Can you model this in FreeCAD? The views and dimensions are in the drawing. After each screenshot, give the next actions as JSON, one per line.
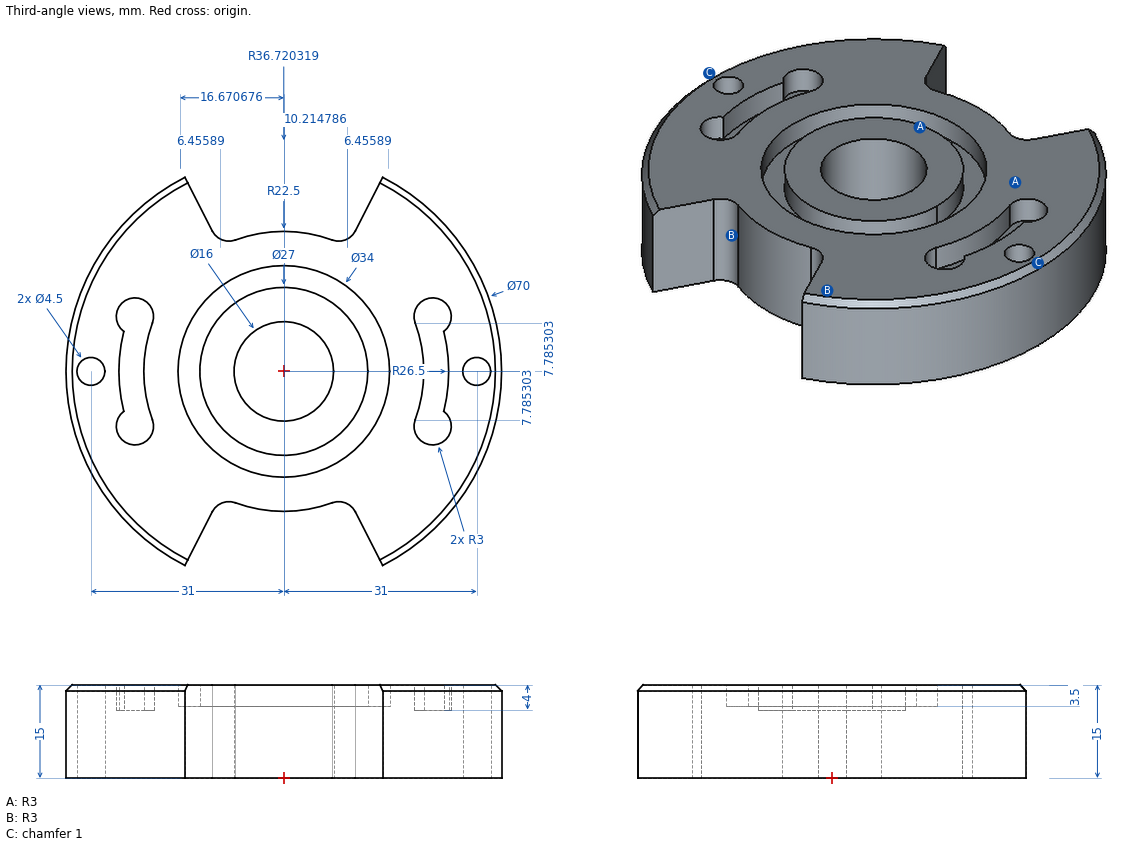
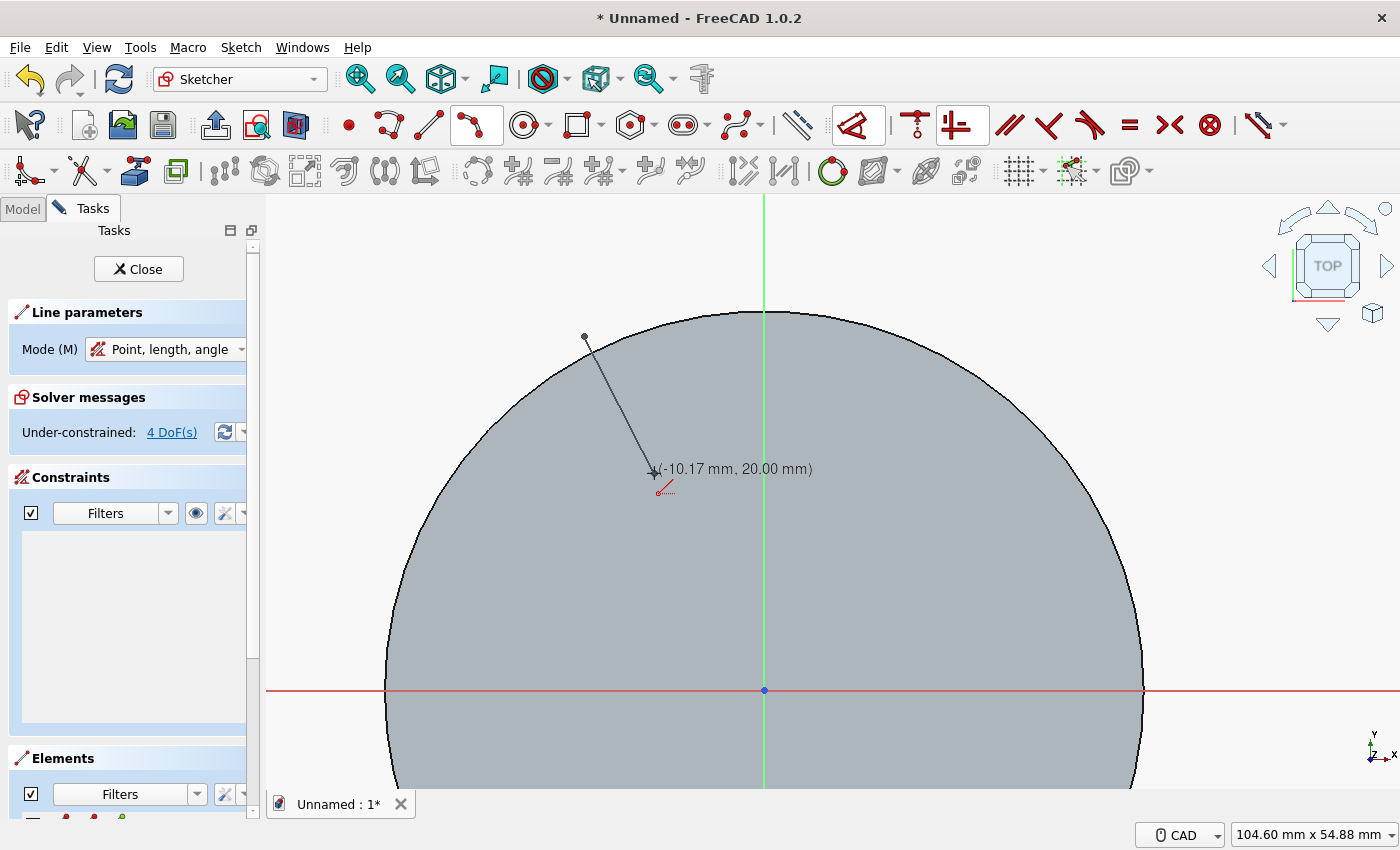
{"action": "left_click", "coordinate": [875, 473]}
{"action": "left_click", "coordinate": [945, 336]}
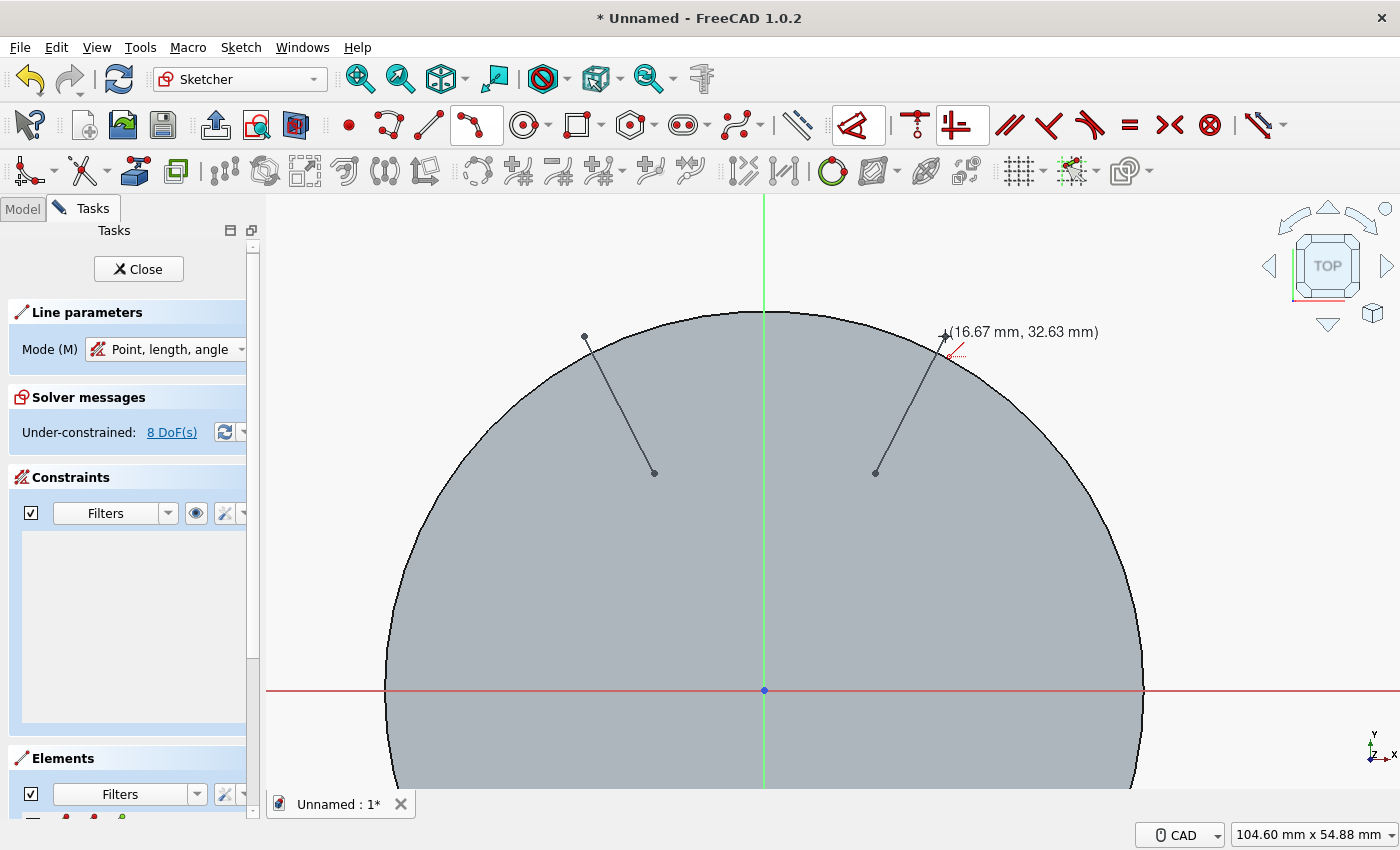
{"action": "key", "text": "g 3 a"}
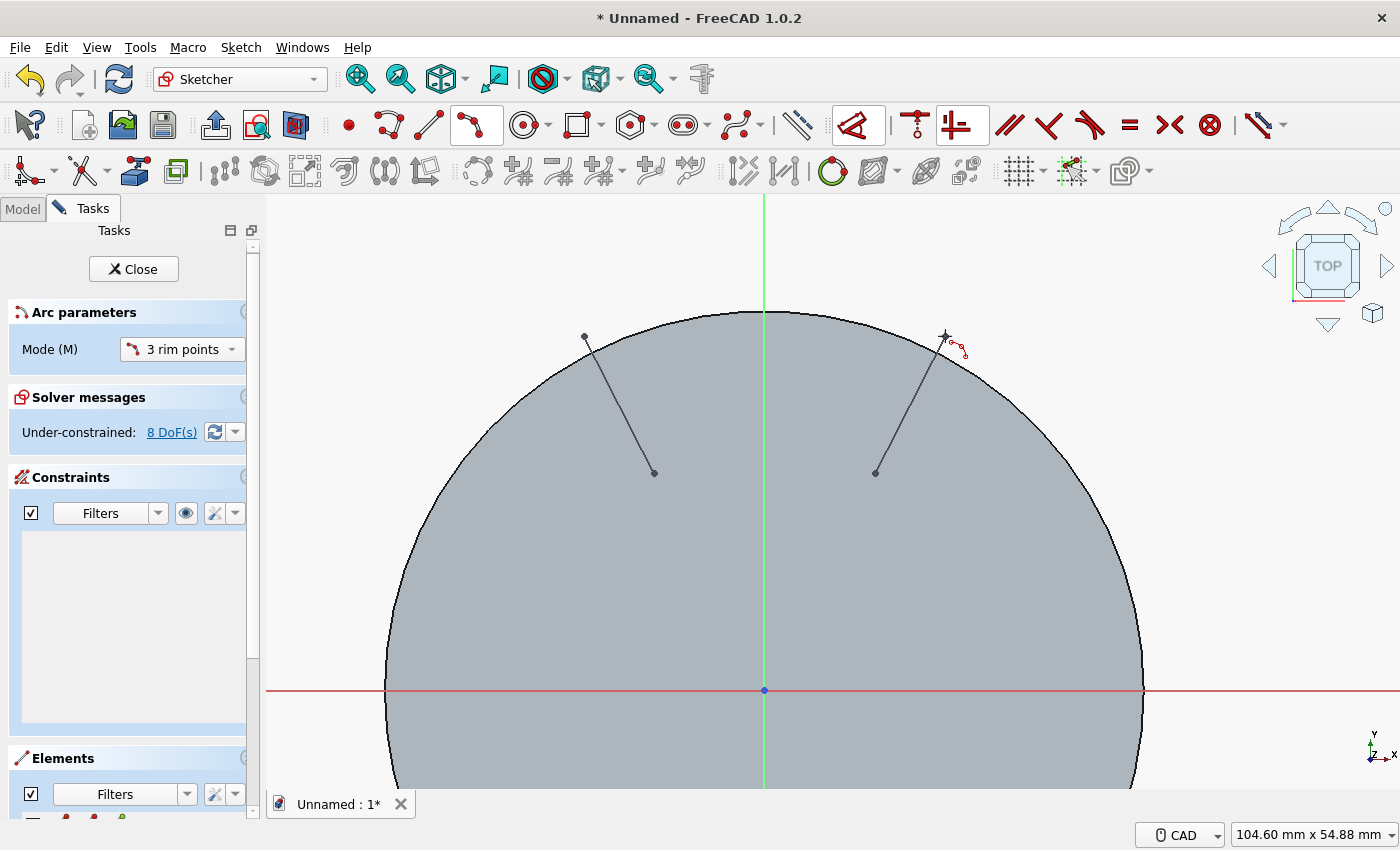
{"action": "left_click", "coordinate": [654, 474]}
{"action": "left_click", "coordinate": [875, 474]}
{"action": "left_click", "coordinate": [787, 448]}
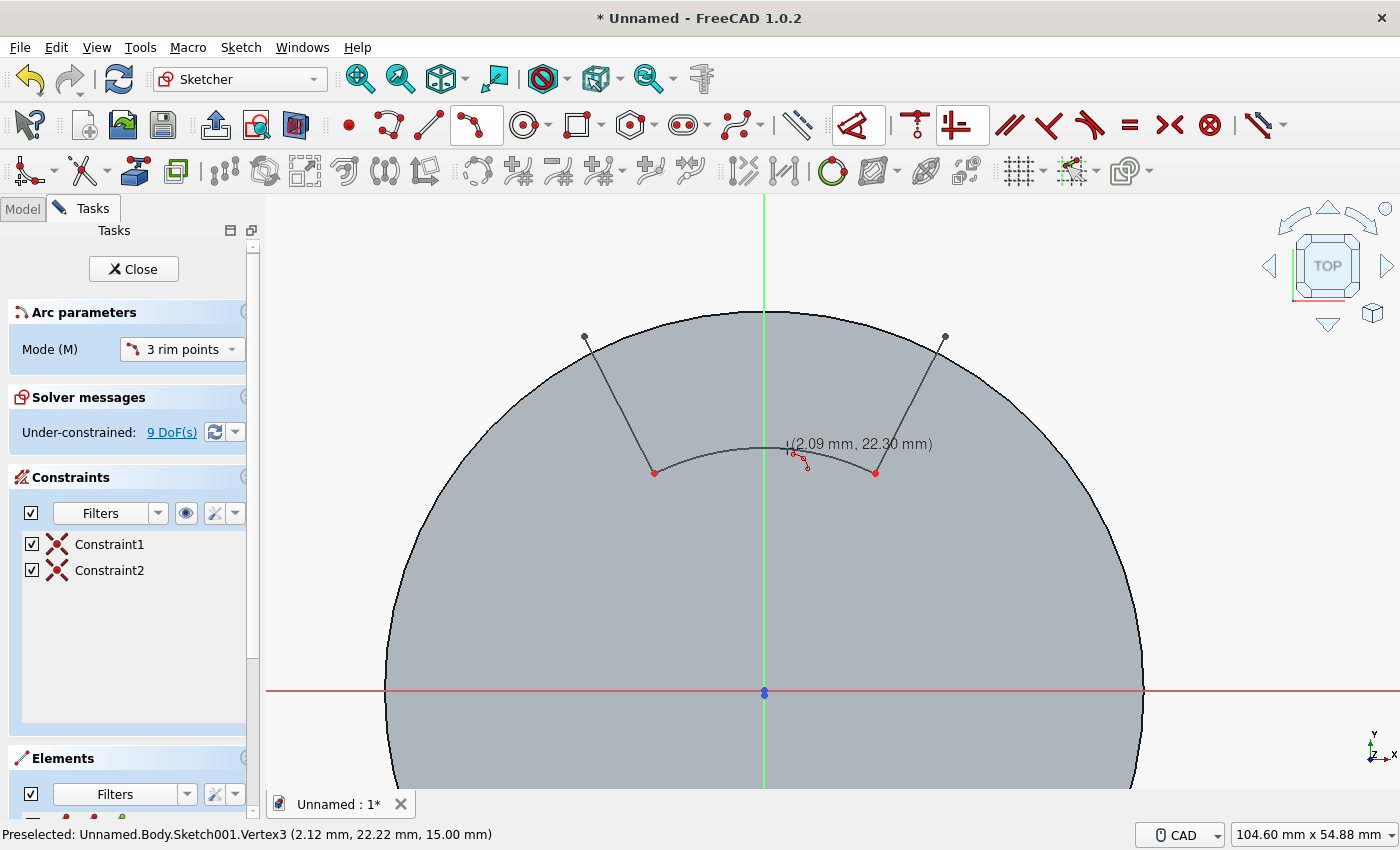
{"action": "left_click", "coordinate": [945, 337]}
{"action": "left_click", "coordinate": [584, 337]}
{"action": "left_click", "coordinate": [802, 294]}
{"action": "key", "text": "Escape"}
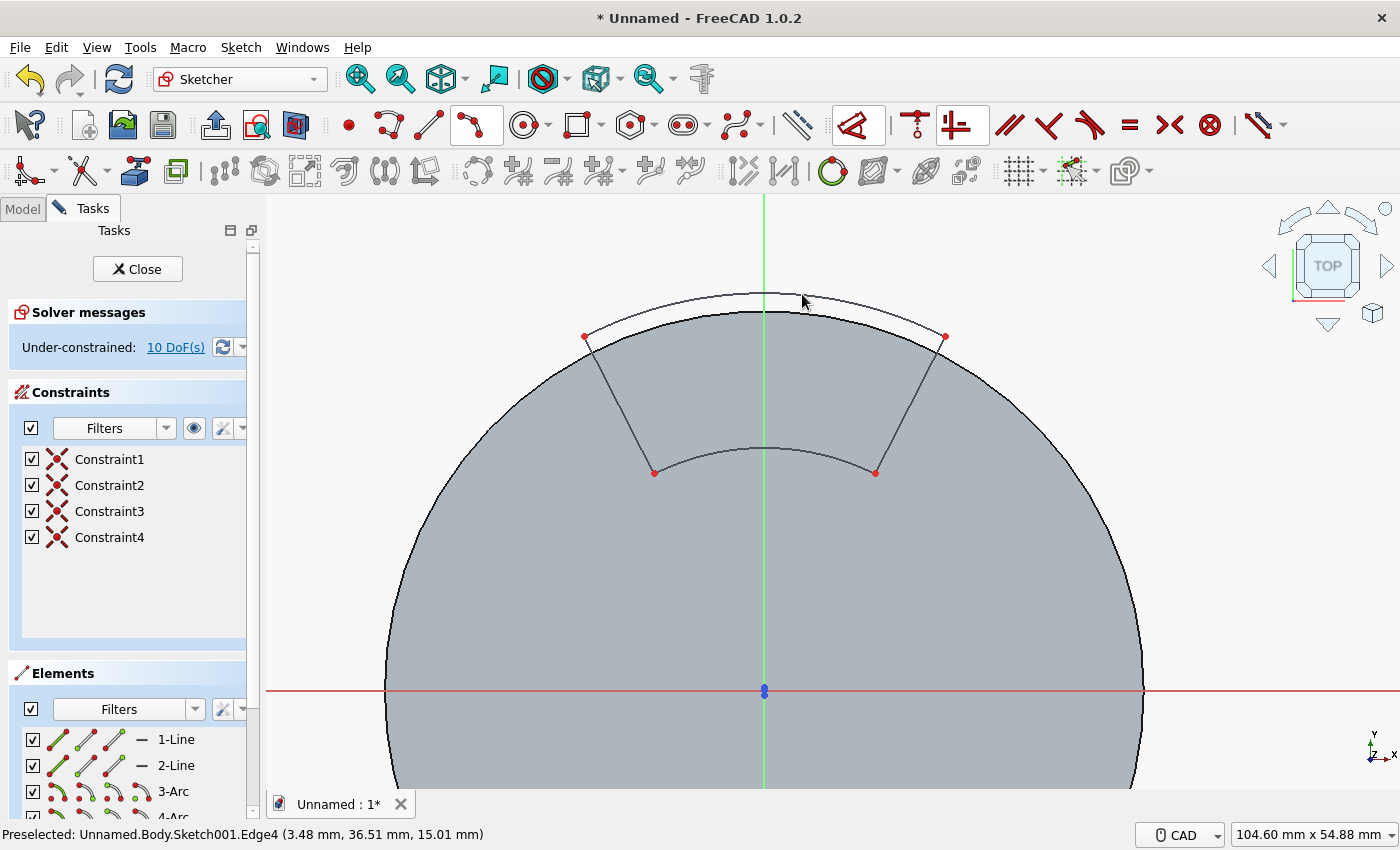
{"action": "left_click", "coordinate": [810, 452]}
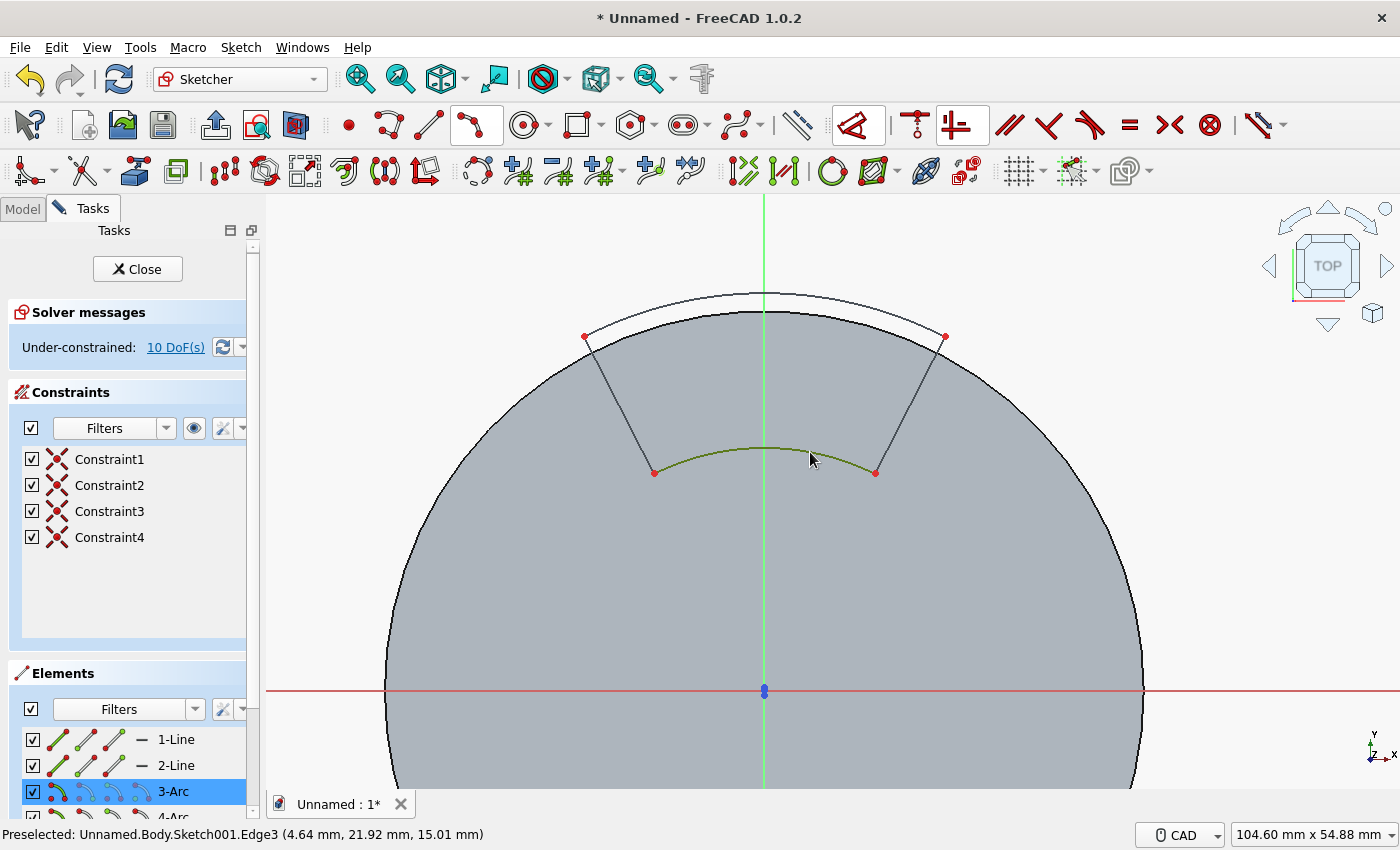
{"action": "left_click", "coordinate": [839, 300]}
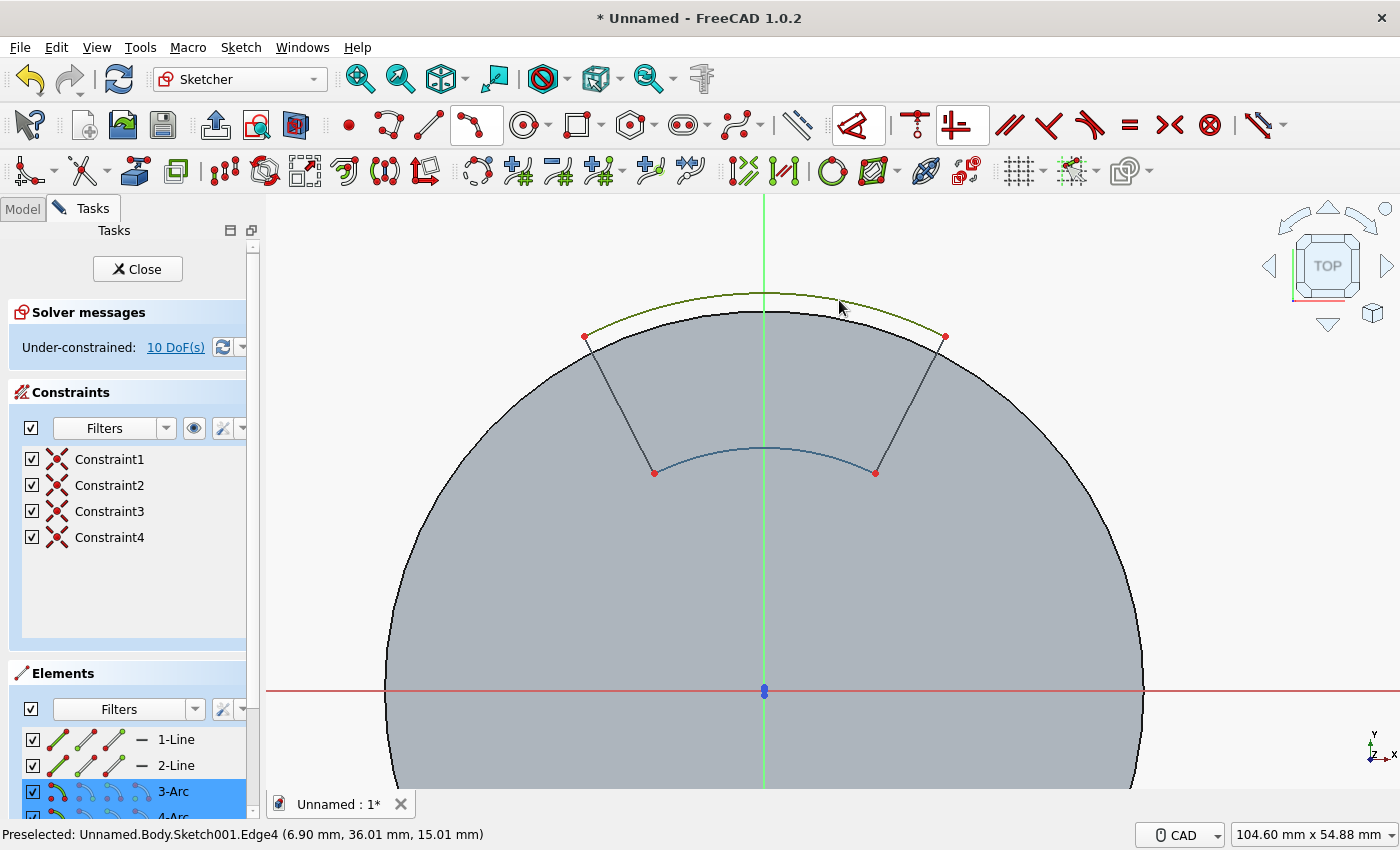
{"action": "left_click", "coordinate": [916, 126]}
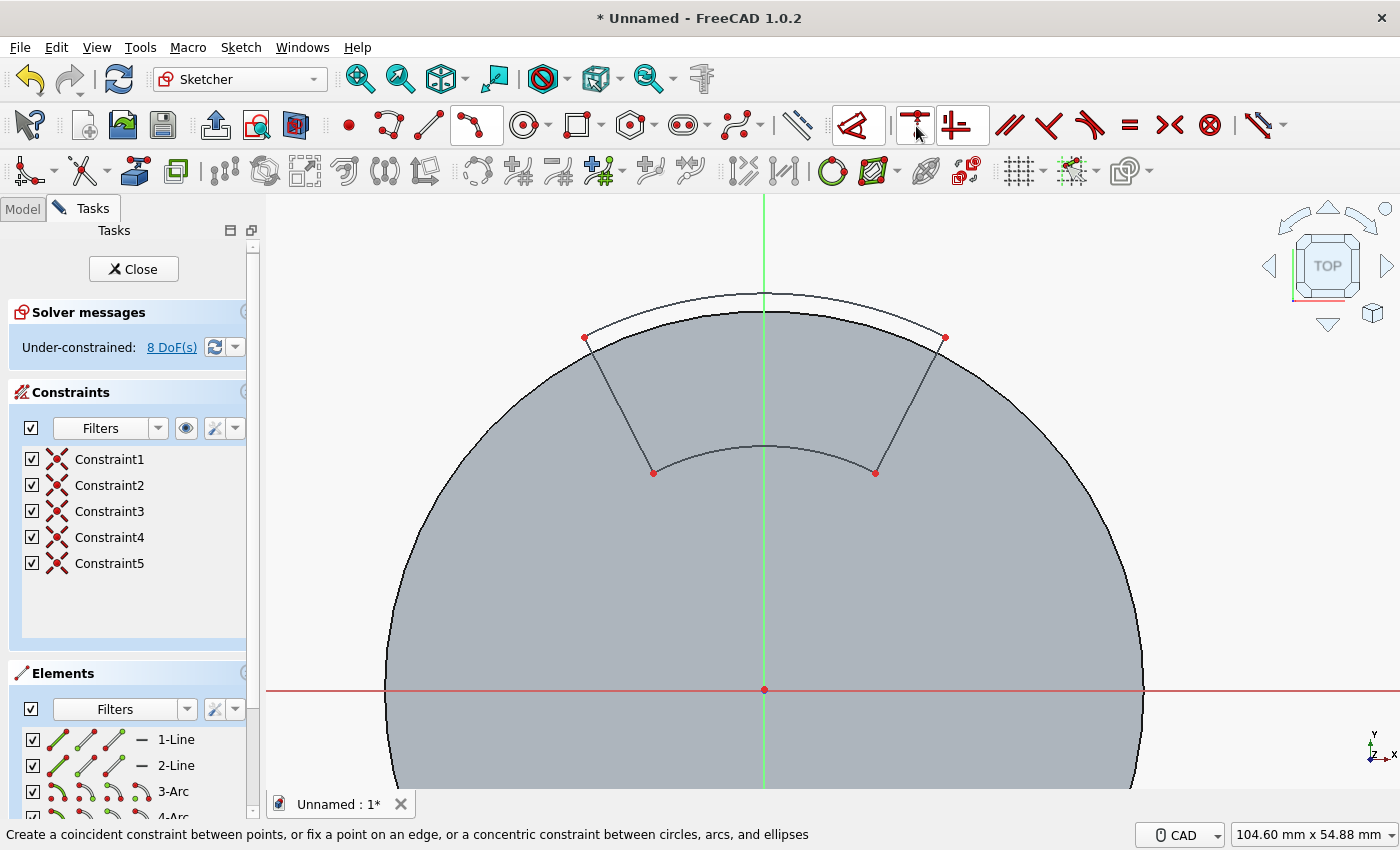
{"action": "left_click_drag", "start_coordinate": [754, 679], "coordinate": [774, 701]}